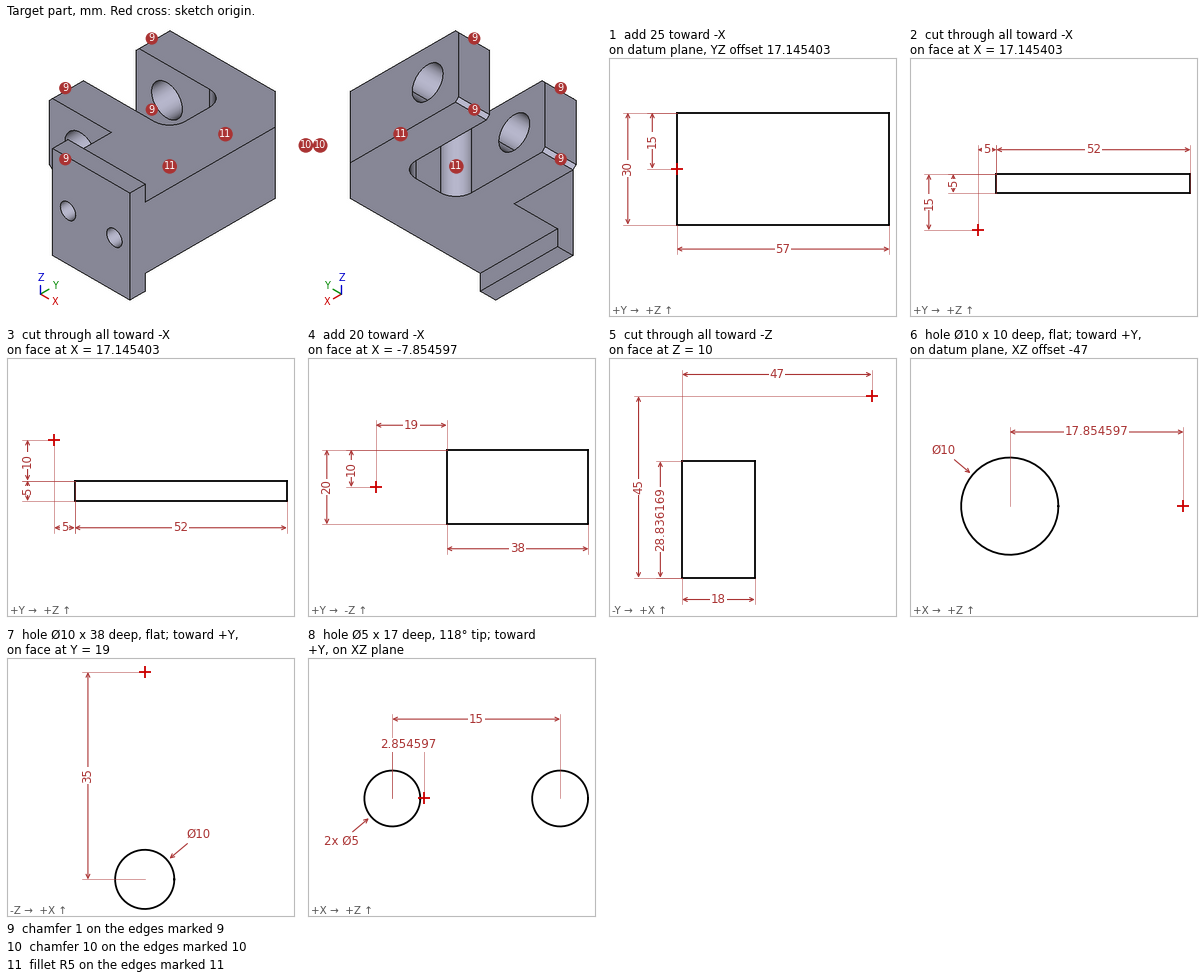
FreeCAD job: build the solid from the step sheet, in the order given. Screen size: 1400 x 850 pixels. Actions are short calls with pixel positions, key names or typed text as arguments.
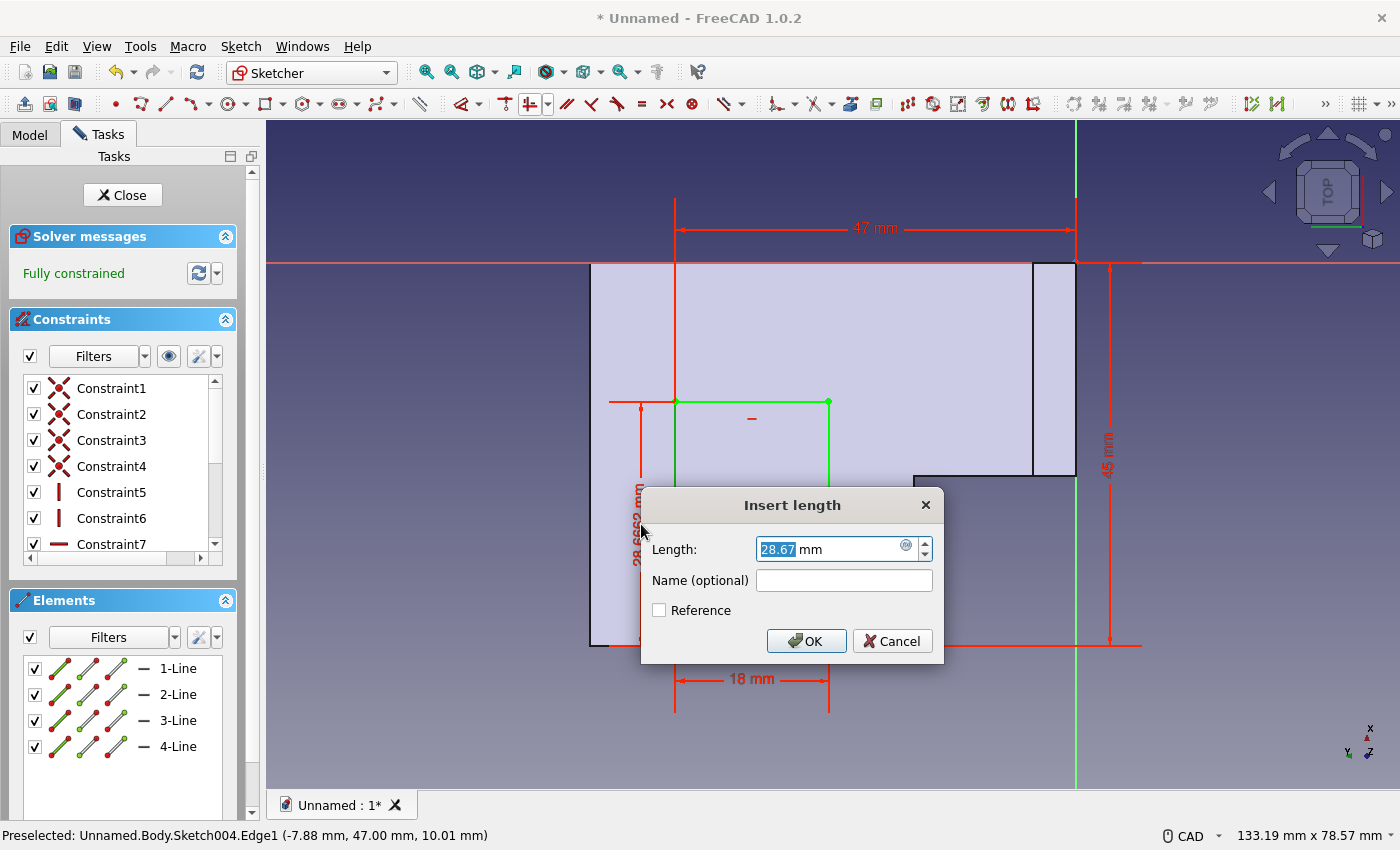
text(28.836169)
key(Return)
key(Escape)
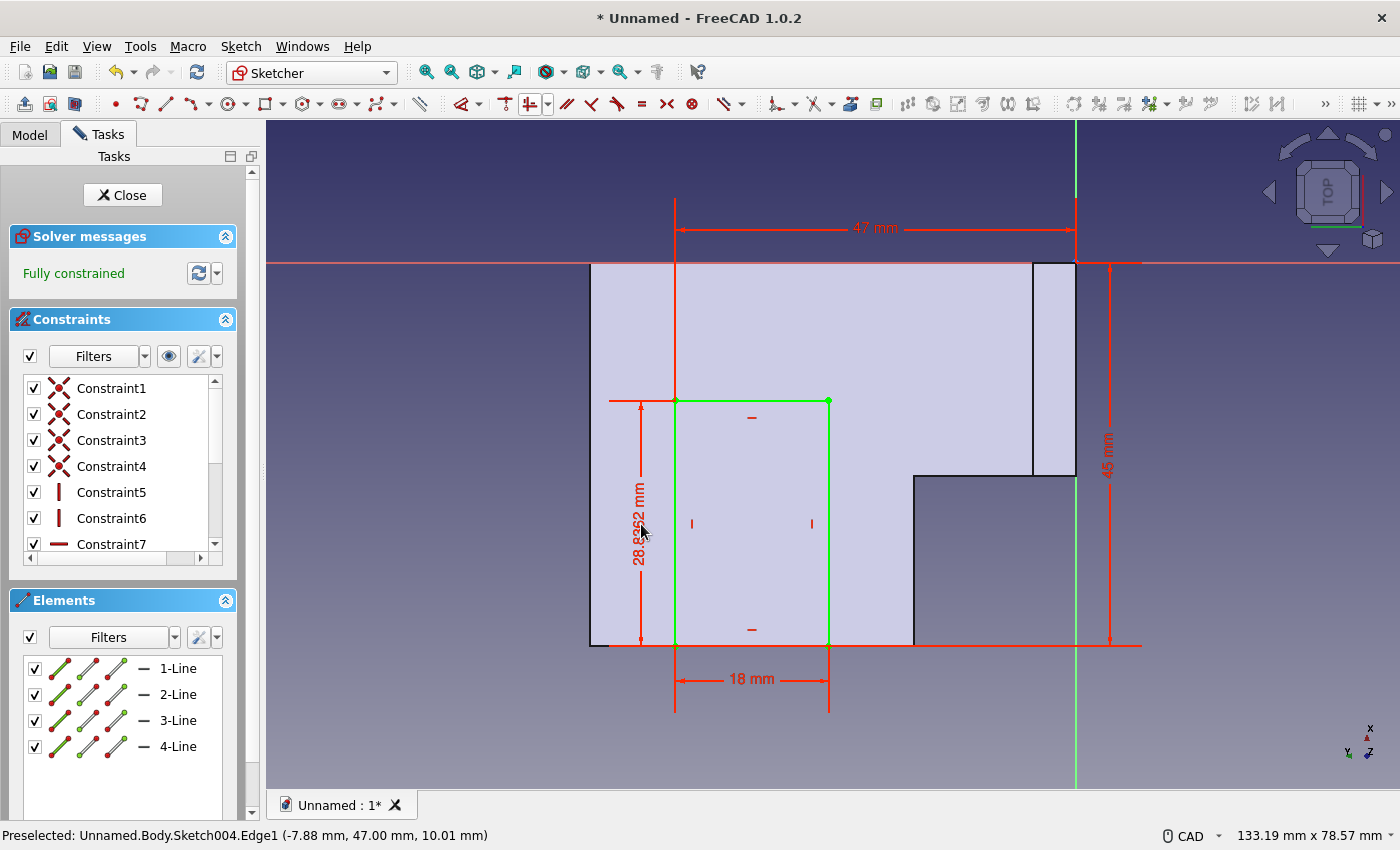
click(123, 195)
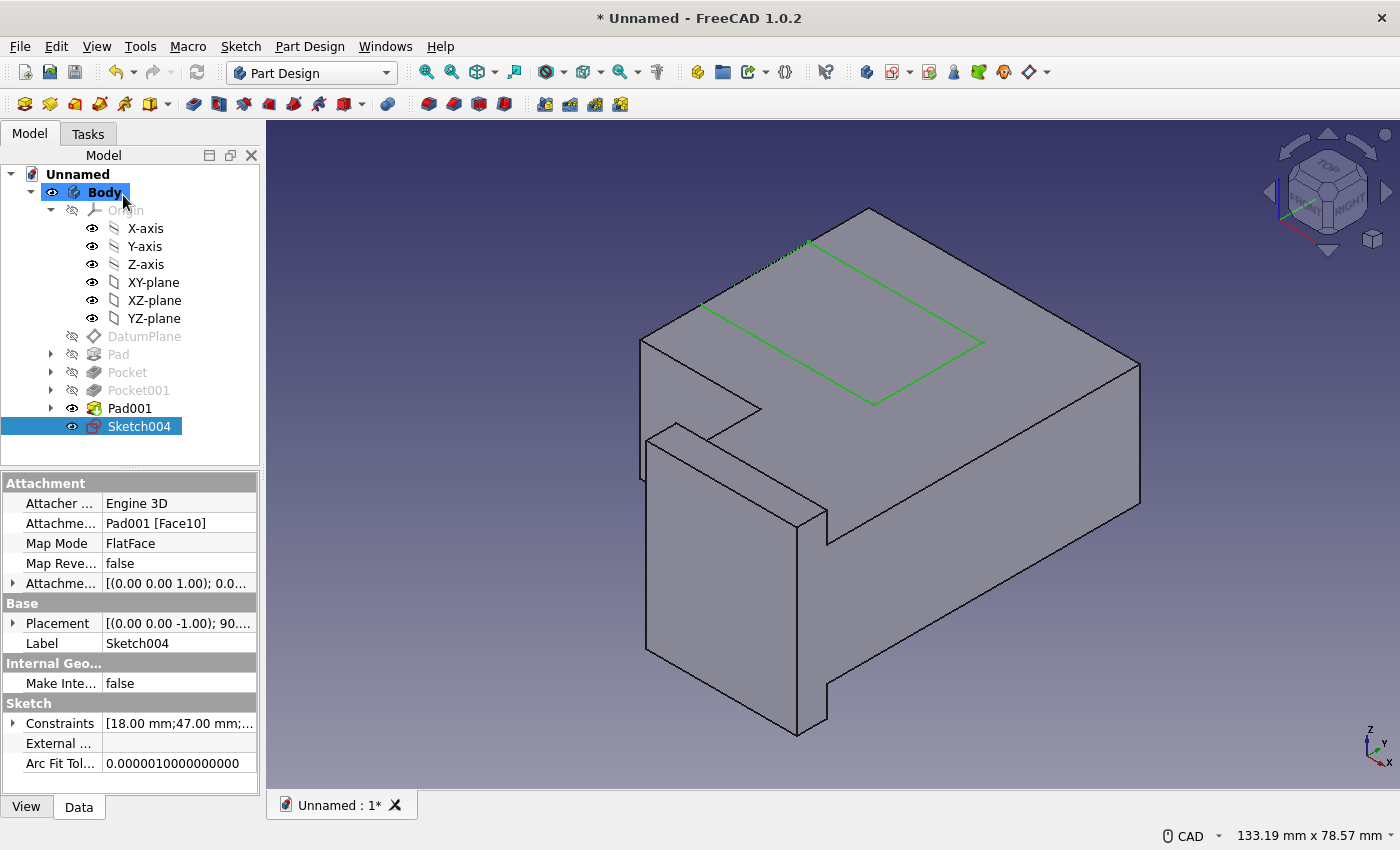
click(194, 104)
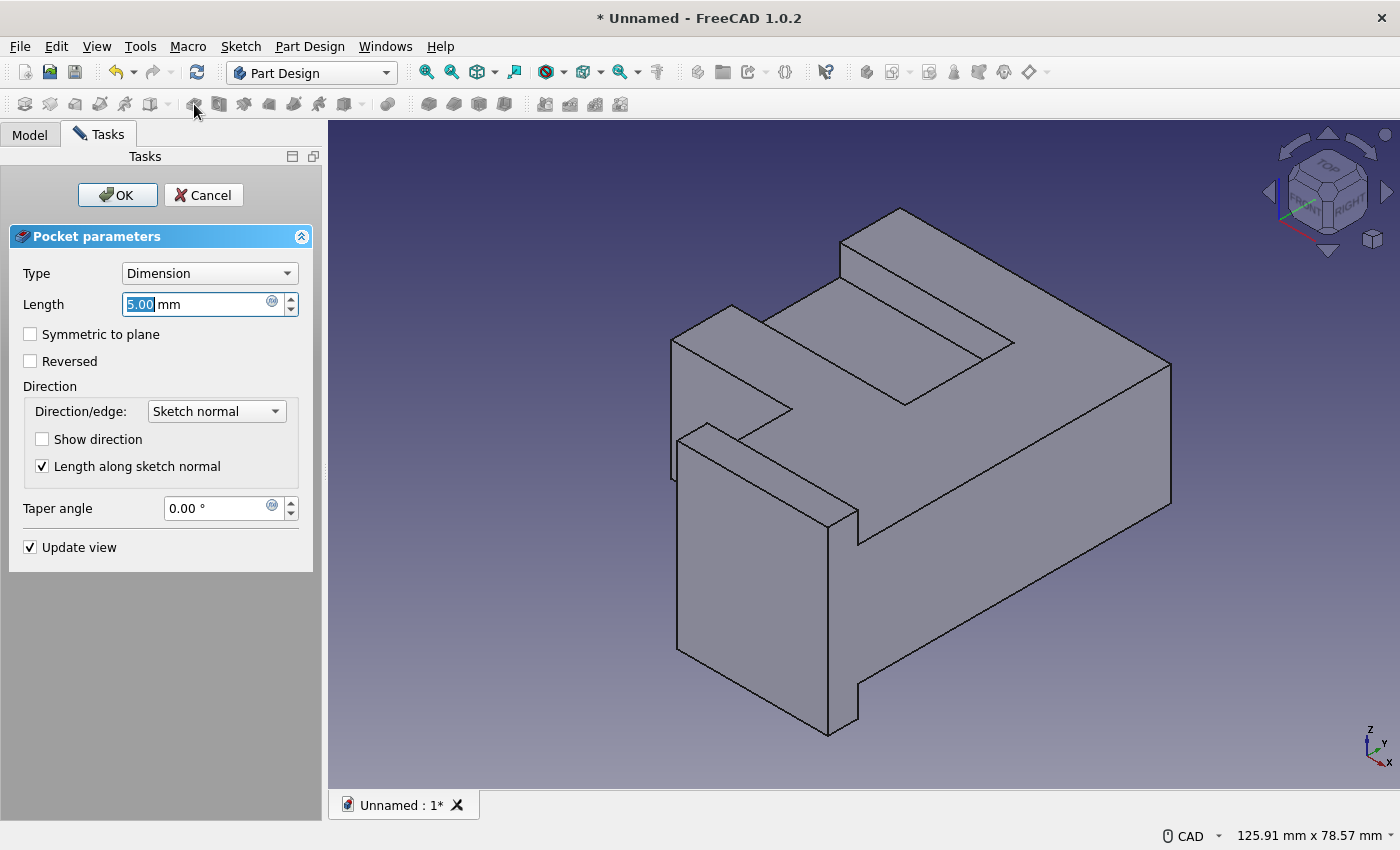
click(210, 274)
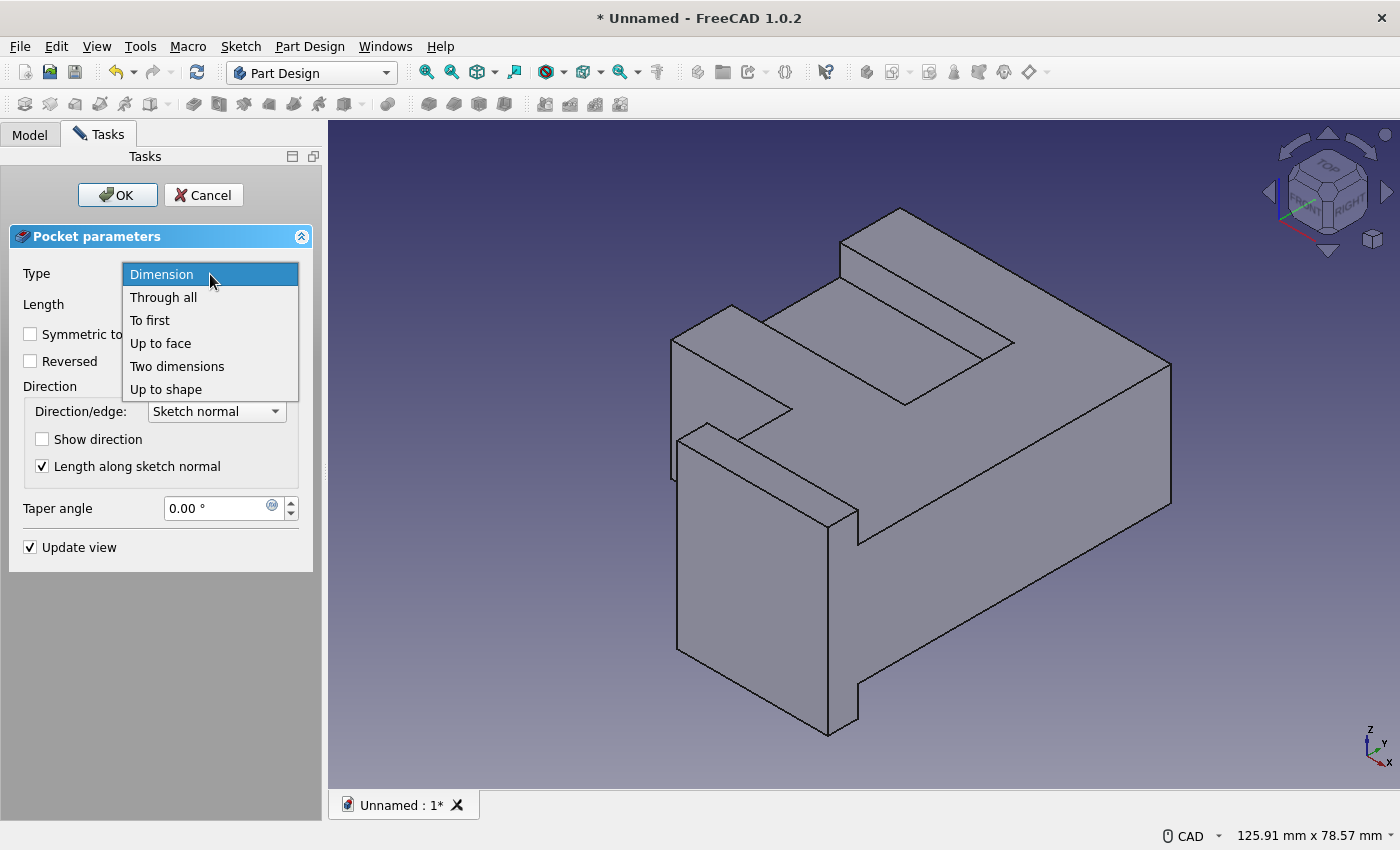
click(208, 298)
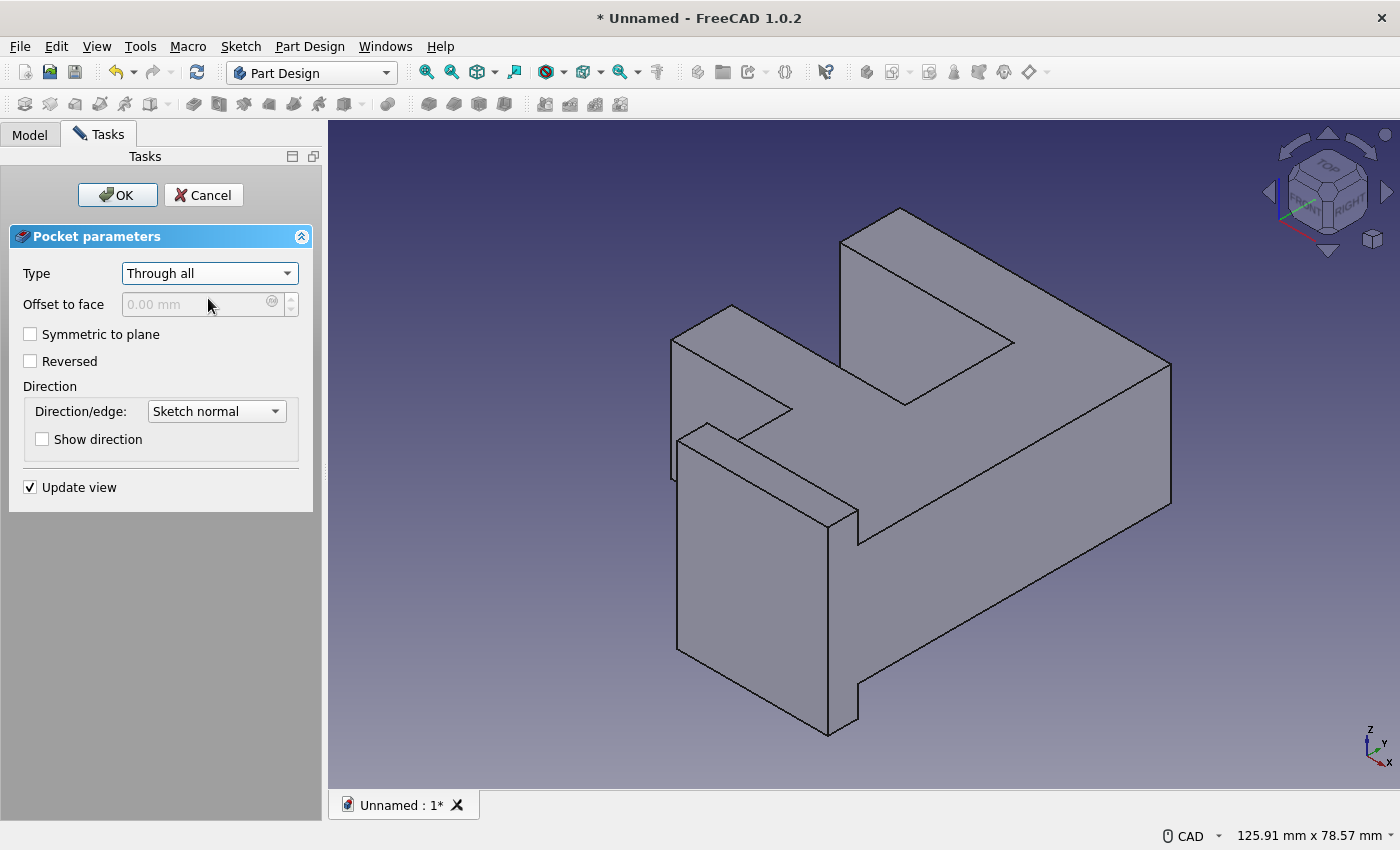
click(118, 195)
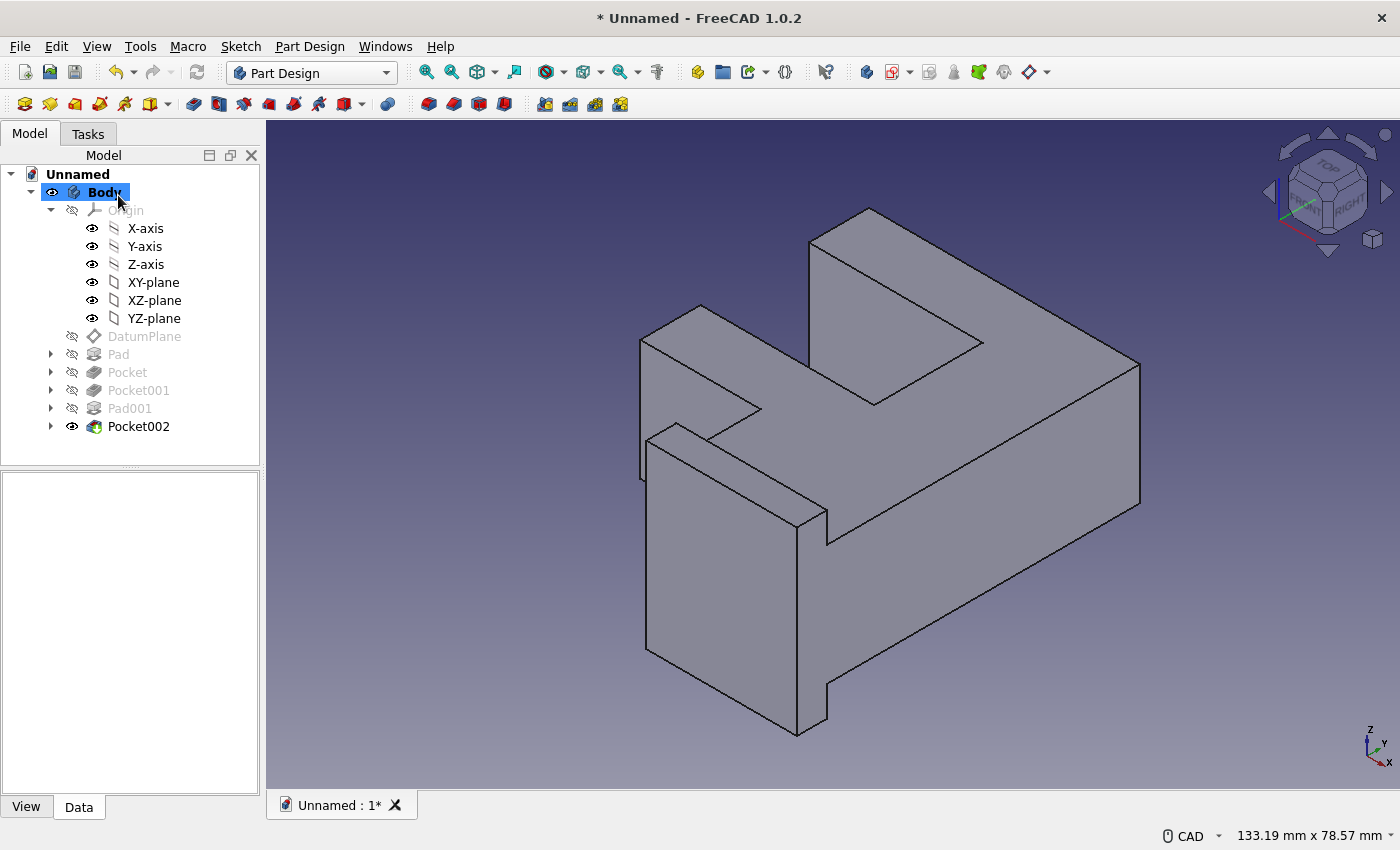
click(137, 300)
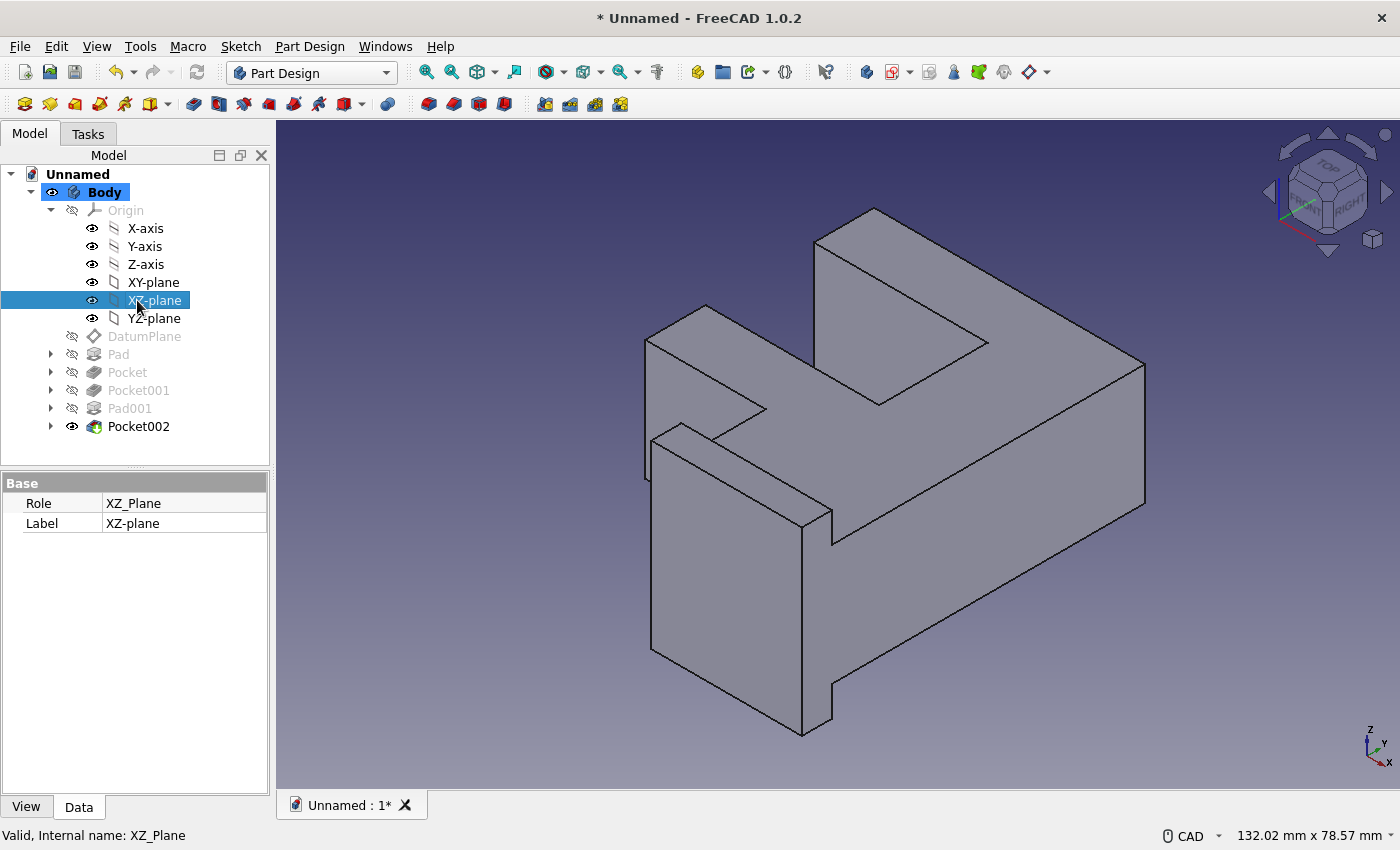
click(1028, 72)